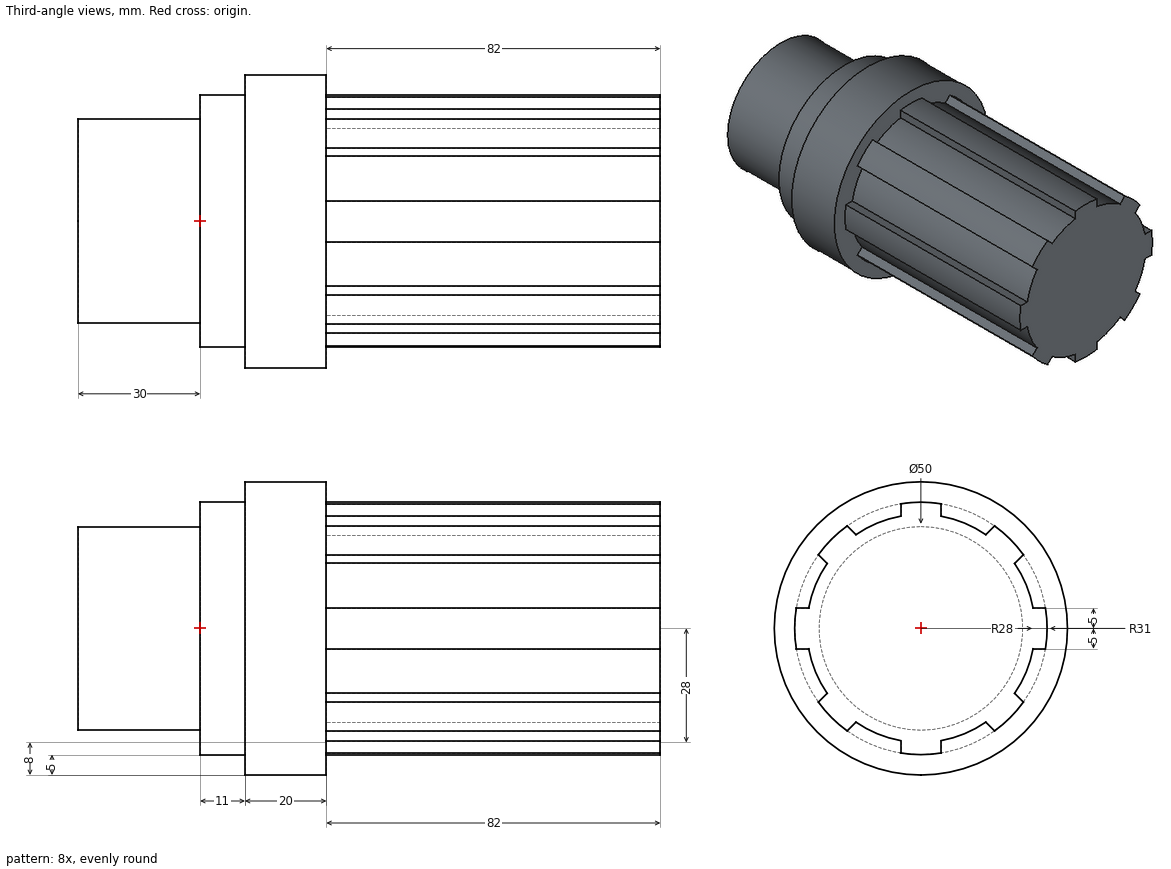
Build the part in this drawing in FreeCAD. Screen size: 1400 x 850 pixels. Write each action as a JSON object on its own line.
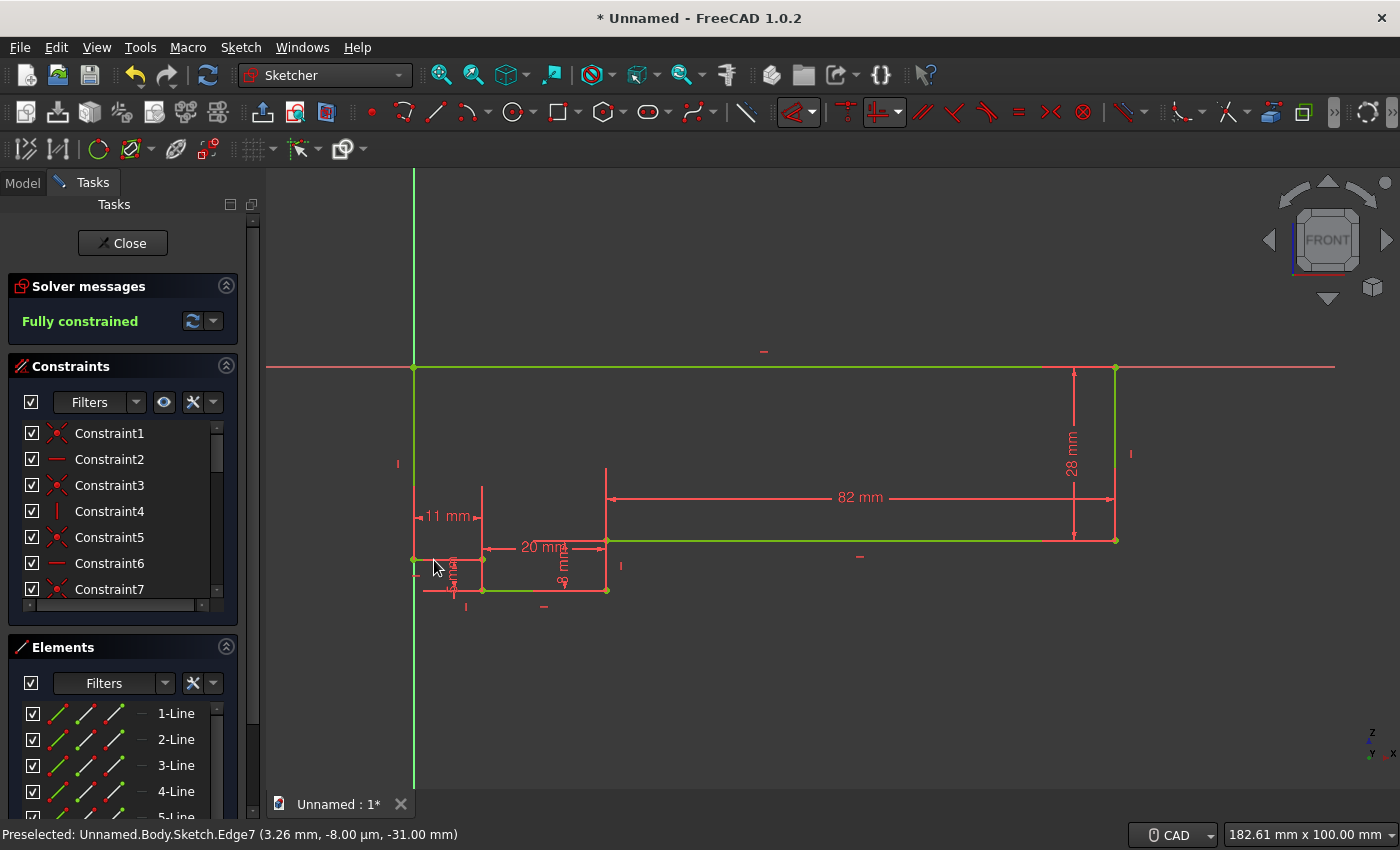
{"action": "left_click", "coordinate": [123, 243]}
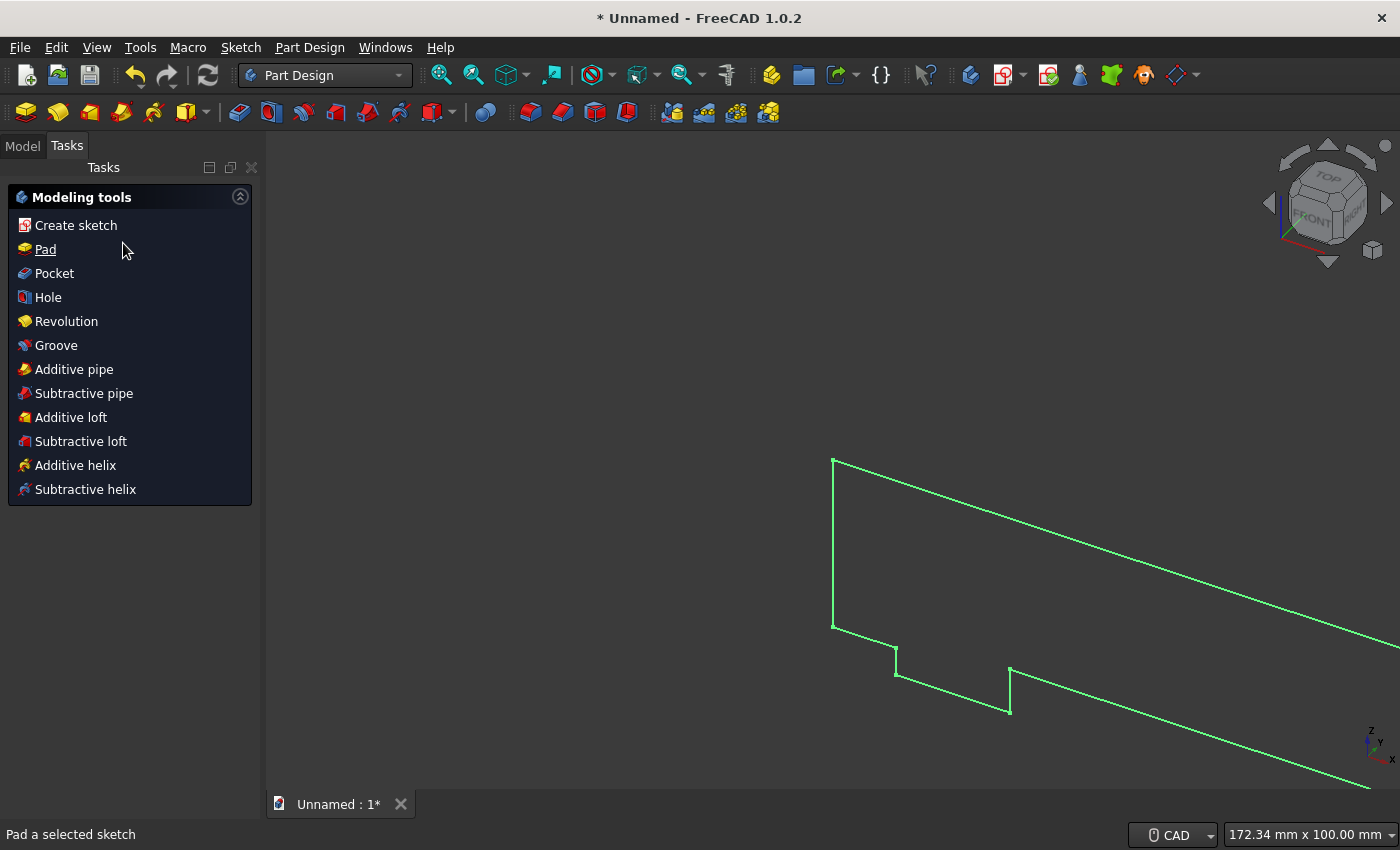
{"action": "left_click", "coordinate": [58, 112]}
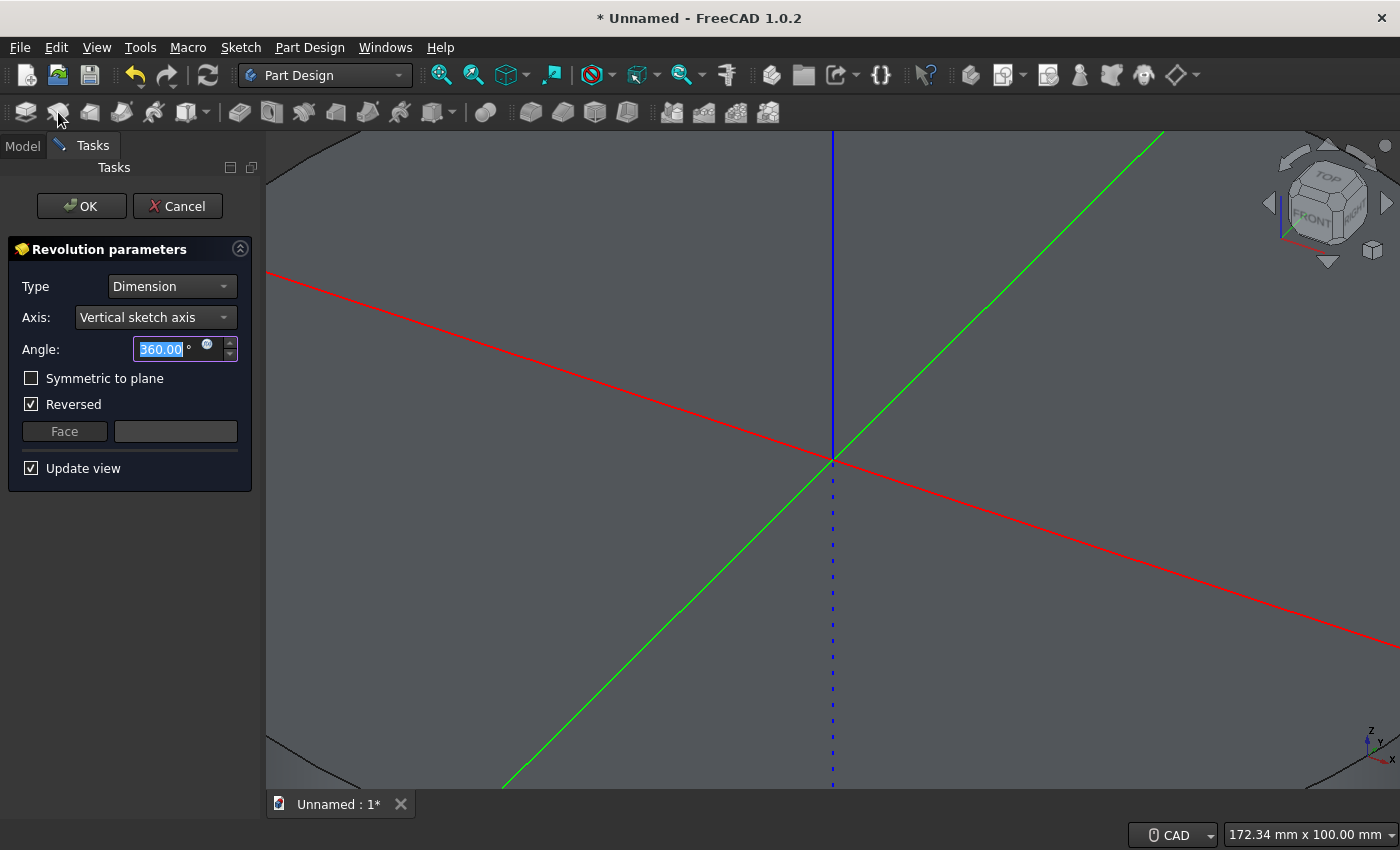
{"action": "left_click", "coordinate": [156, 318]}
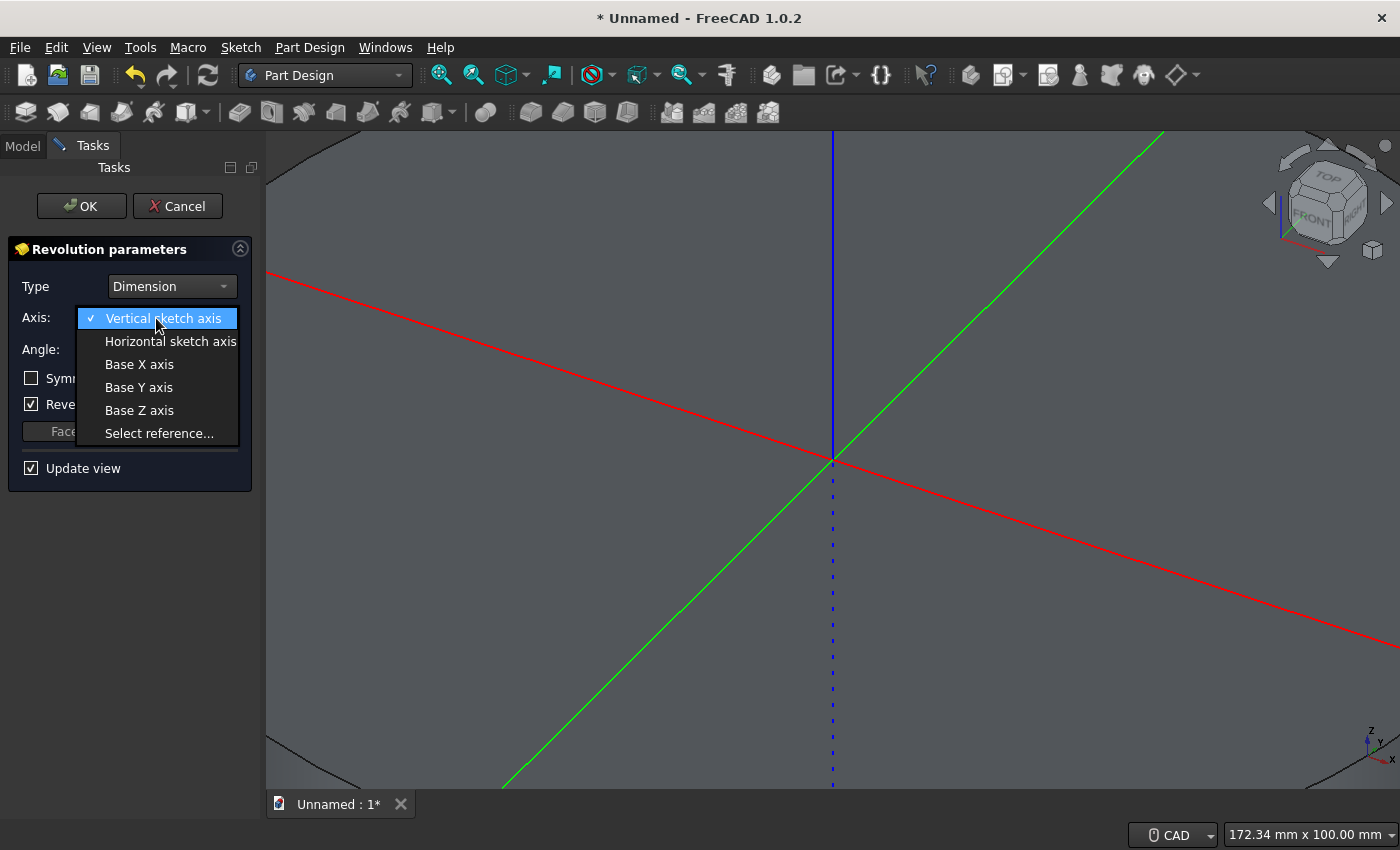
{"action": "left_click", "coordinate": [156, 342]}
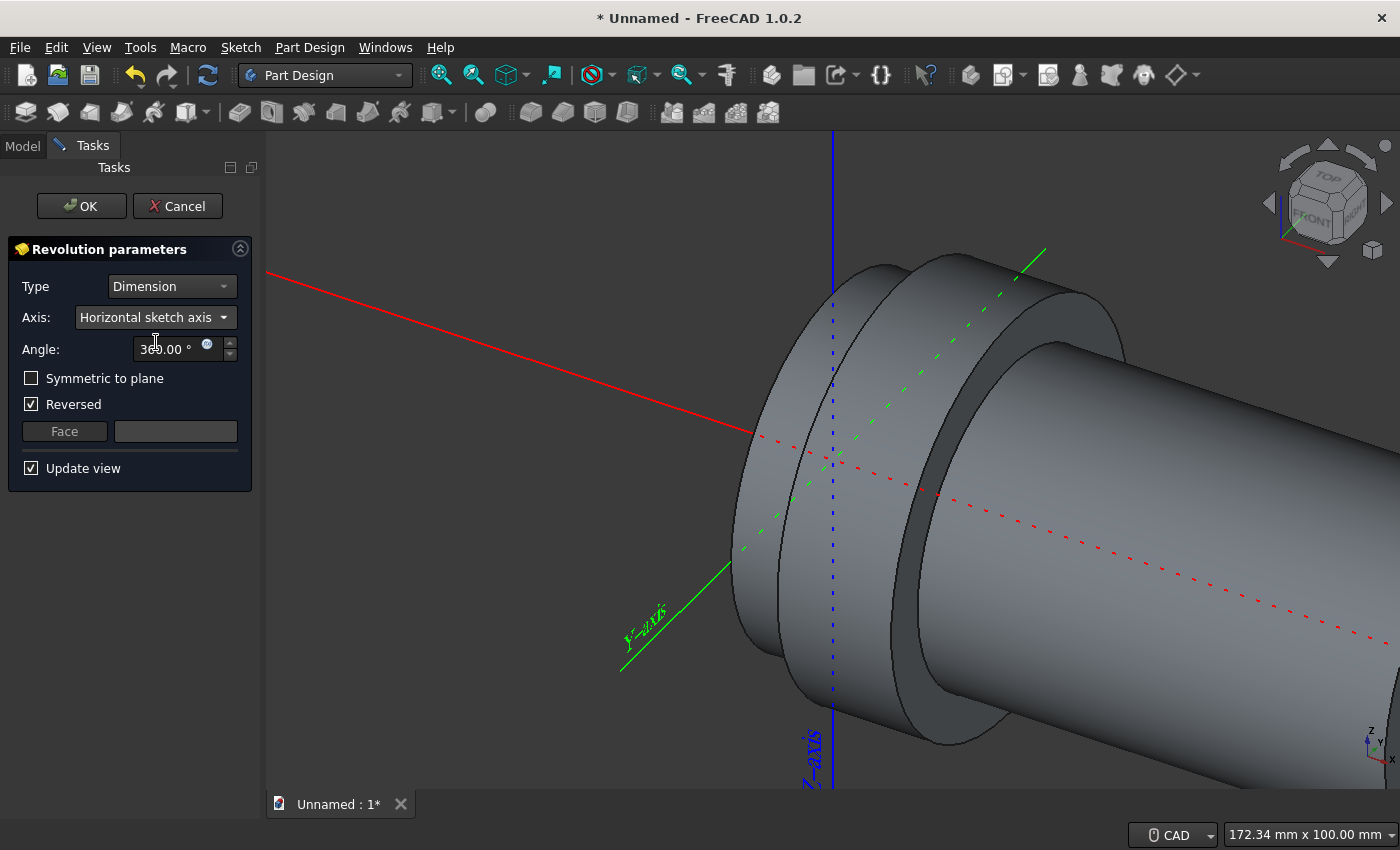
{"action": "left_click", "coordinate": [82, 206]}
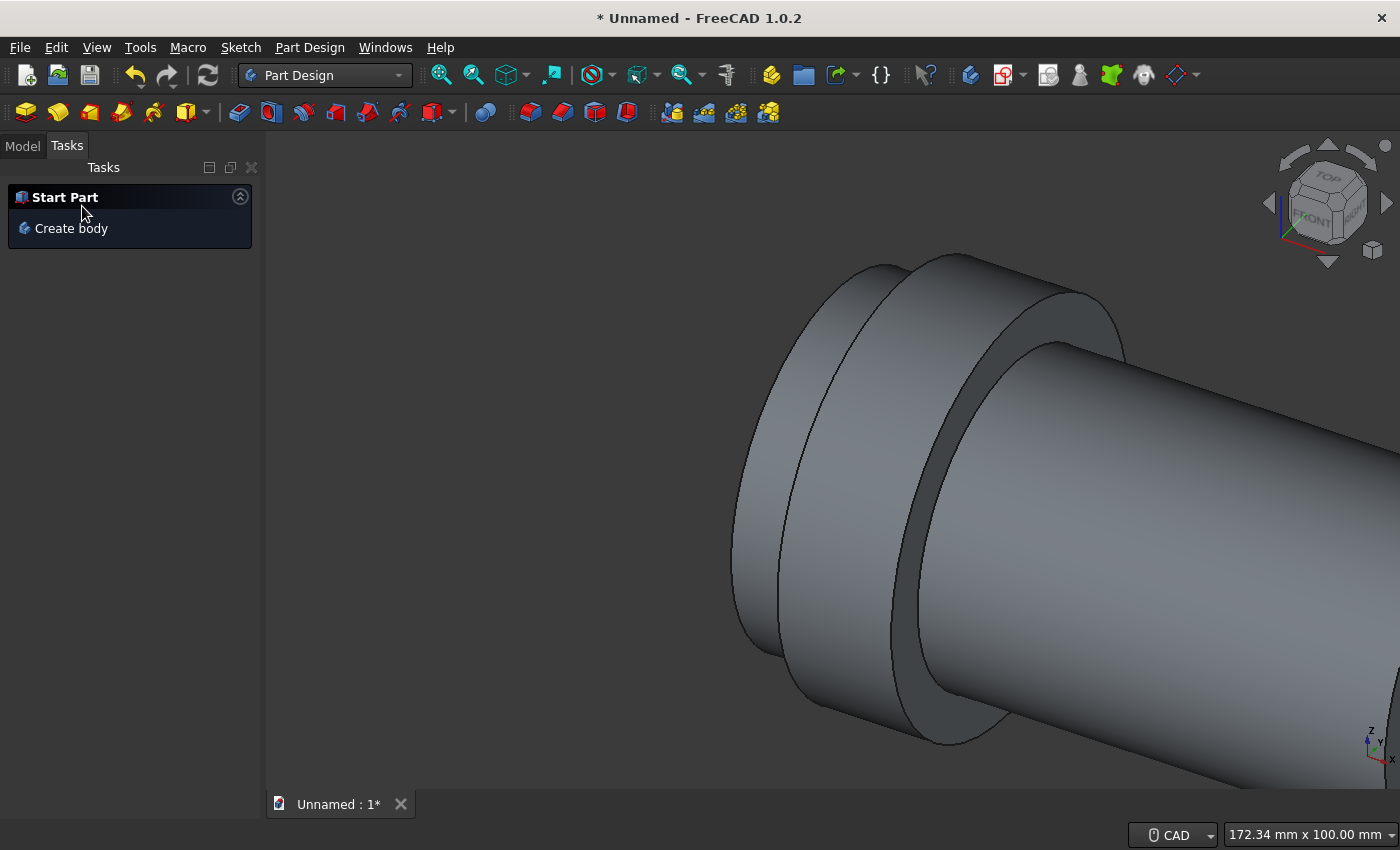
{"action": "key", "text": "v f"}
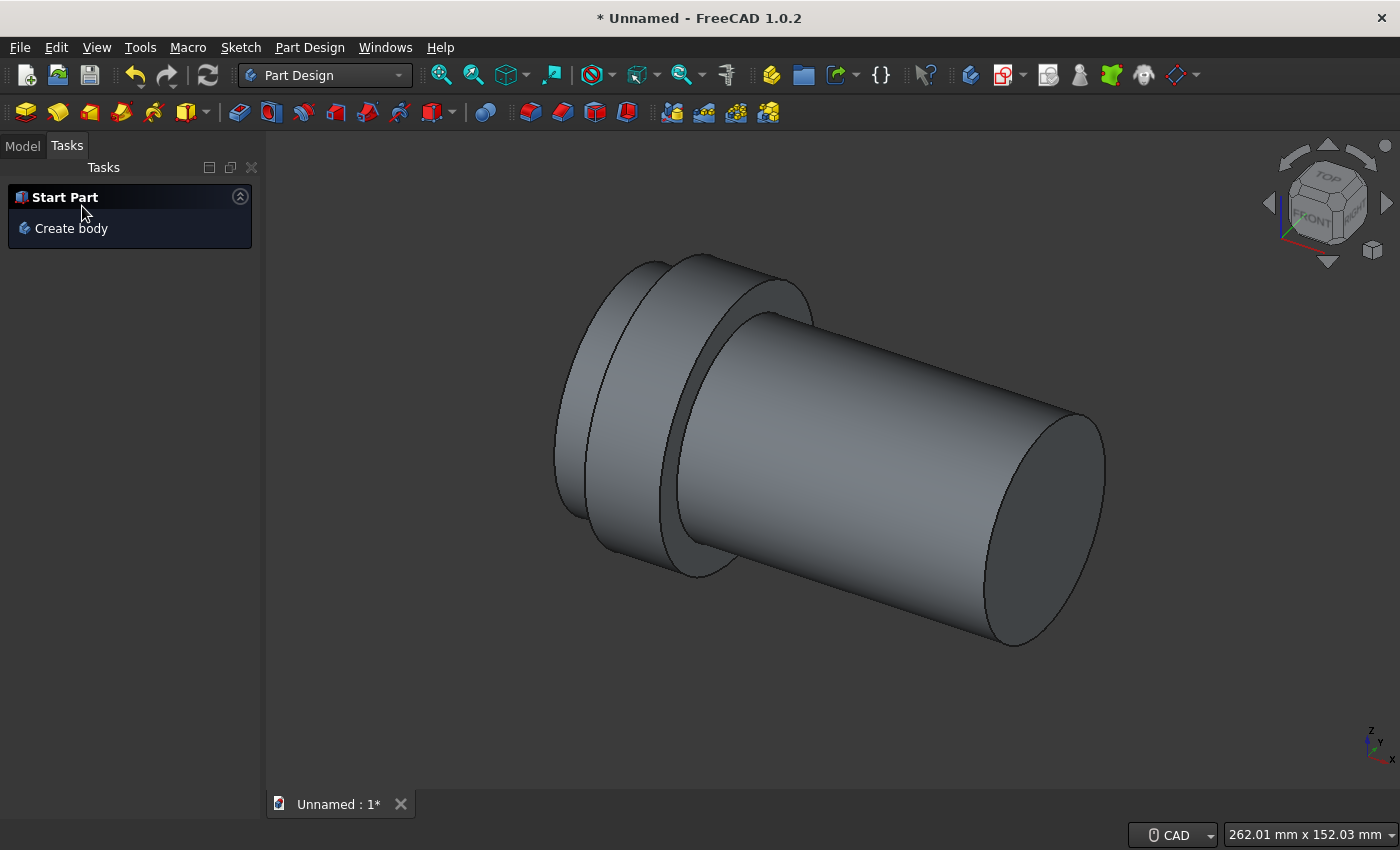
{"action": "left_click", "coordinate": [1045, 529]}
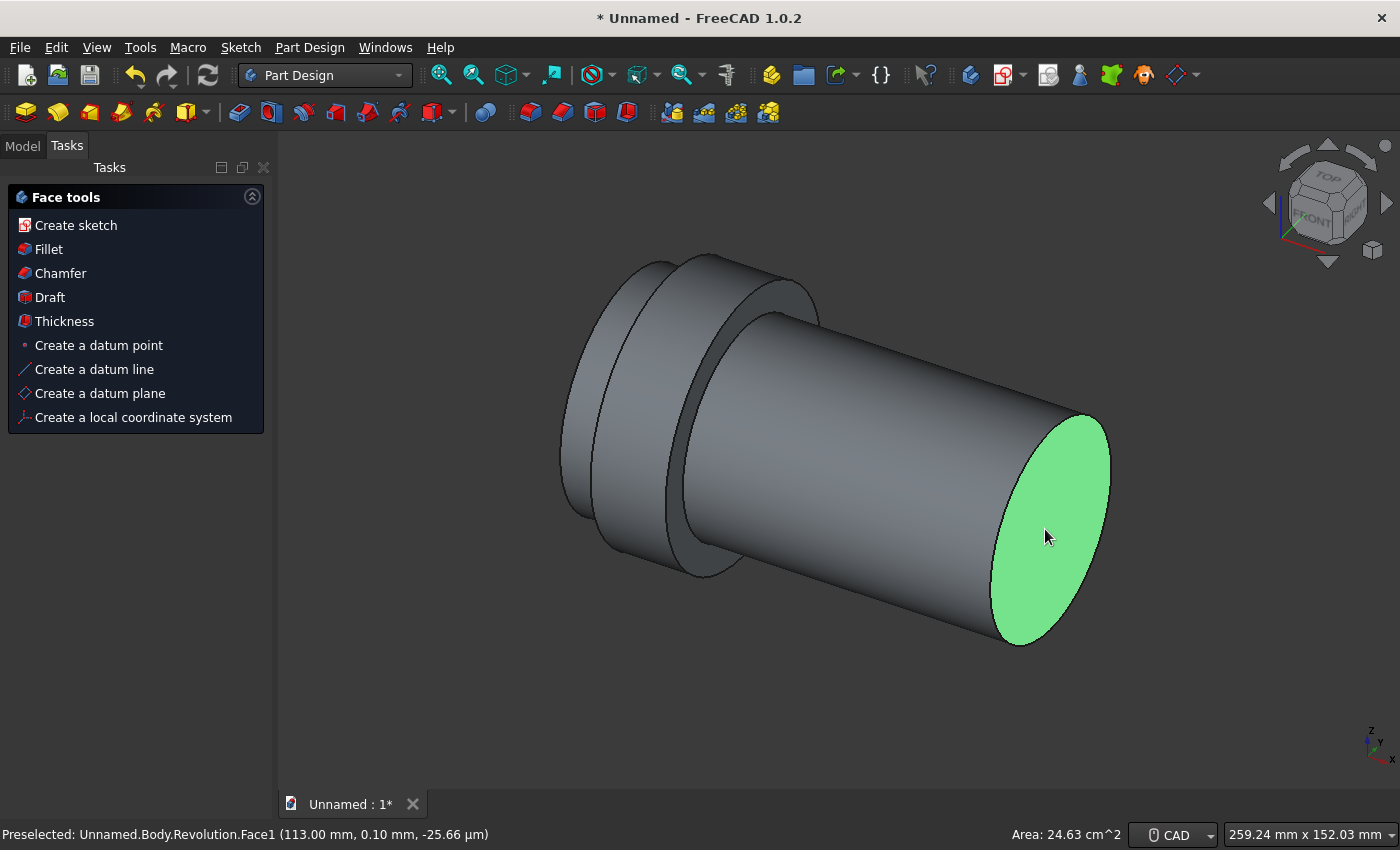
{"action": "left_click", "coordinate": [1004, 76]}